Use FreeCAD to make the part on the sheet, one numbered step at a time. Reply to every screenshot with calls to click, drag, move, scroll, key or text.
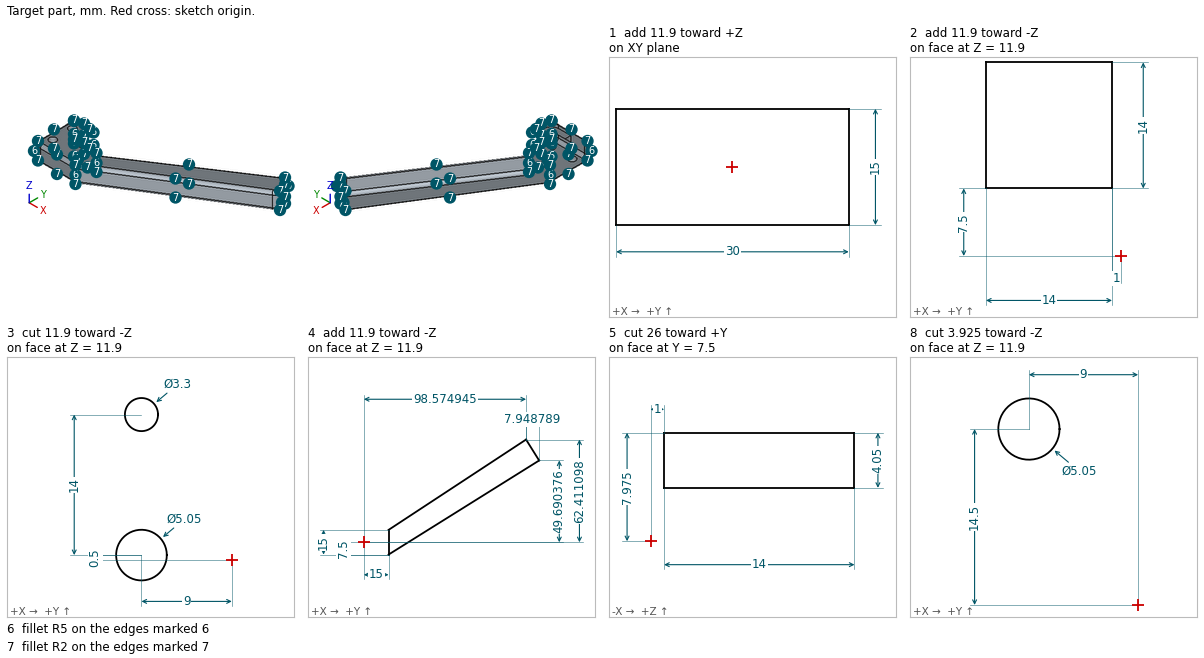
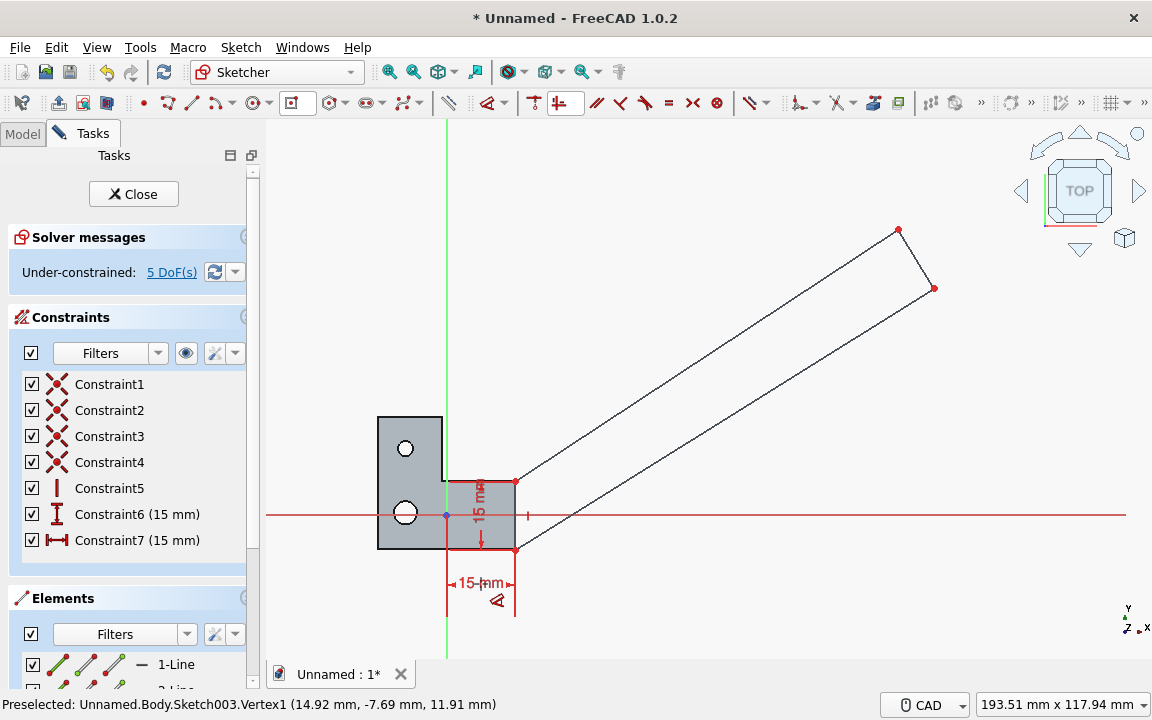
click(515, 550)
click(413, 533)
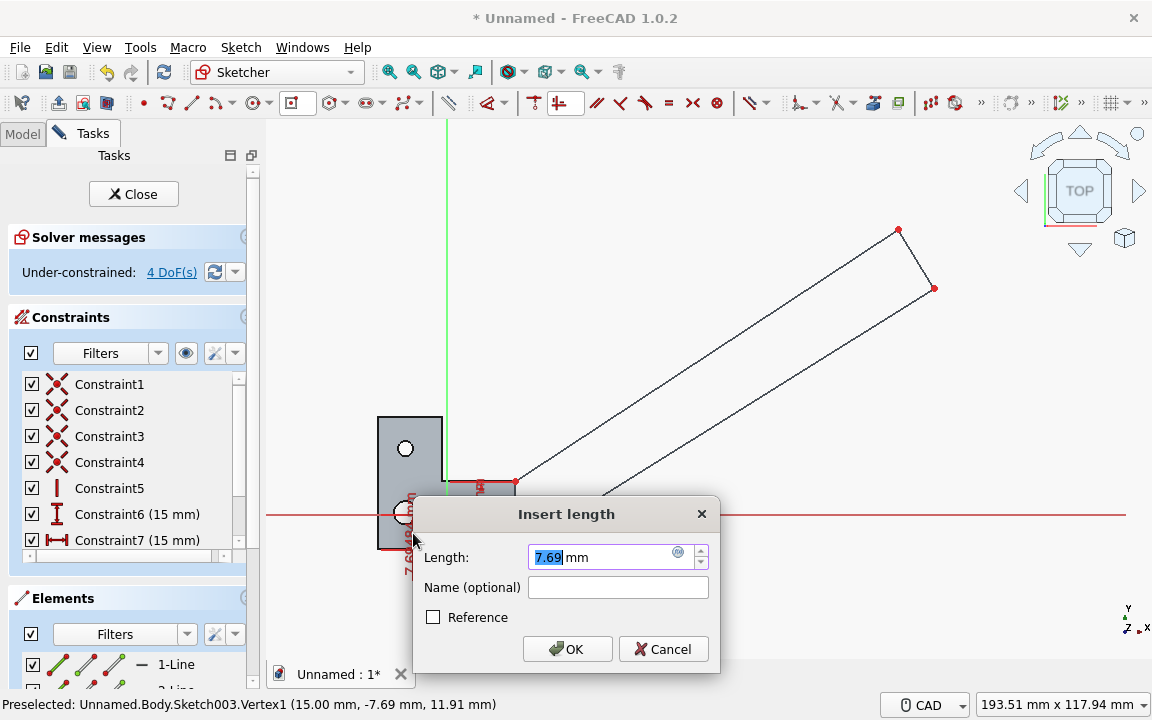
text(7.5)
key(Return)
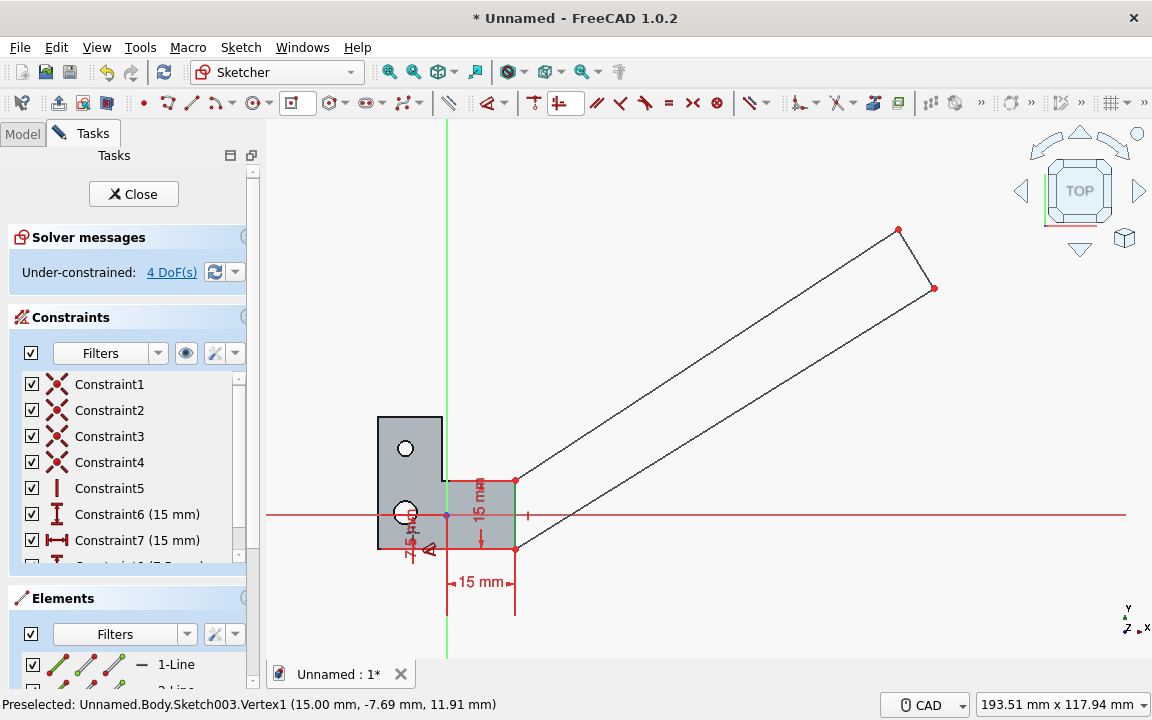
click(923, 271)
click(916, 196)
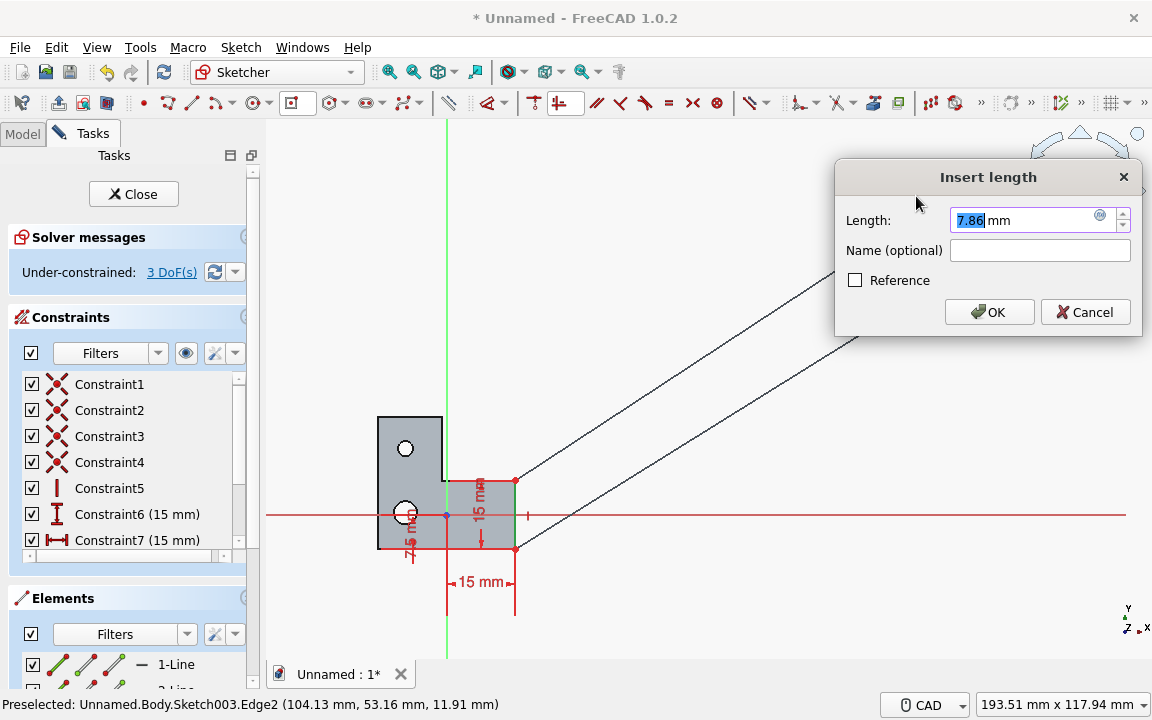
text(7.948789)
key(Return)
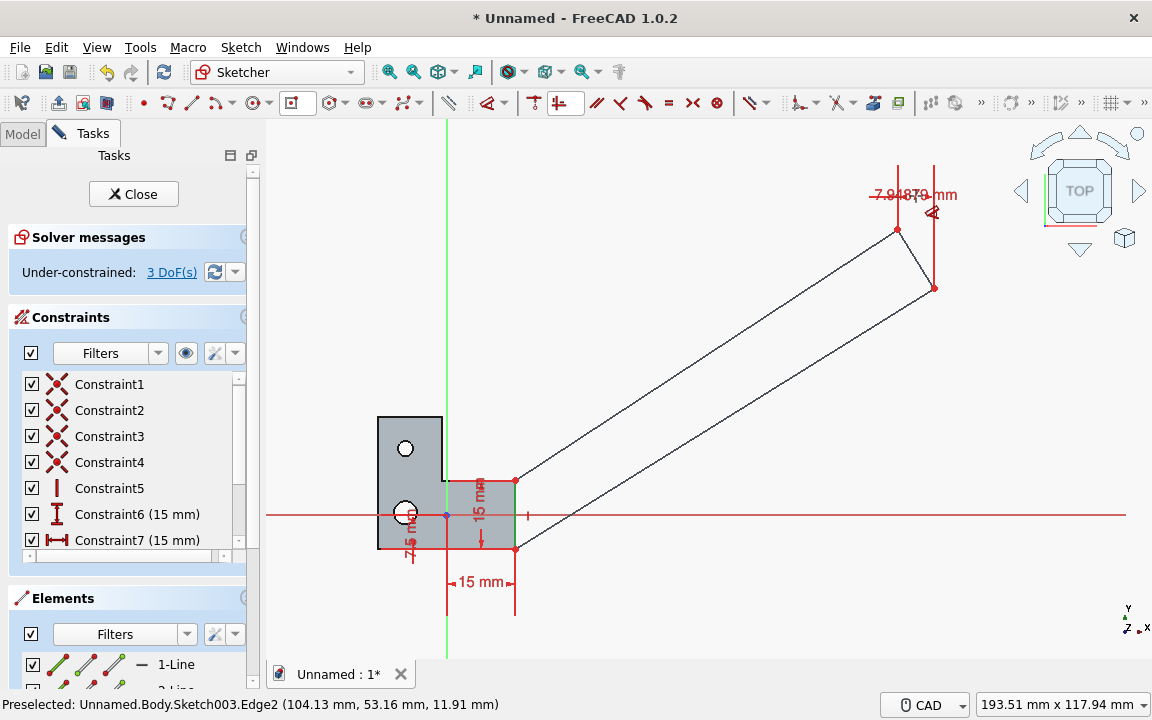
click(934, 289)
click(413, 402)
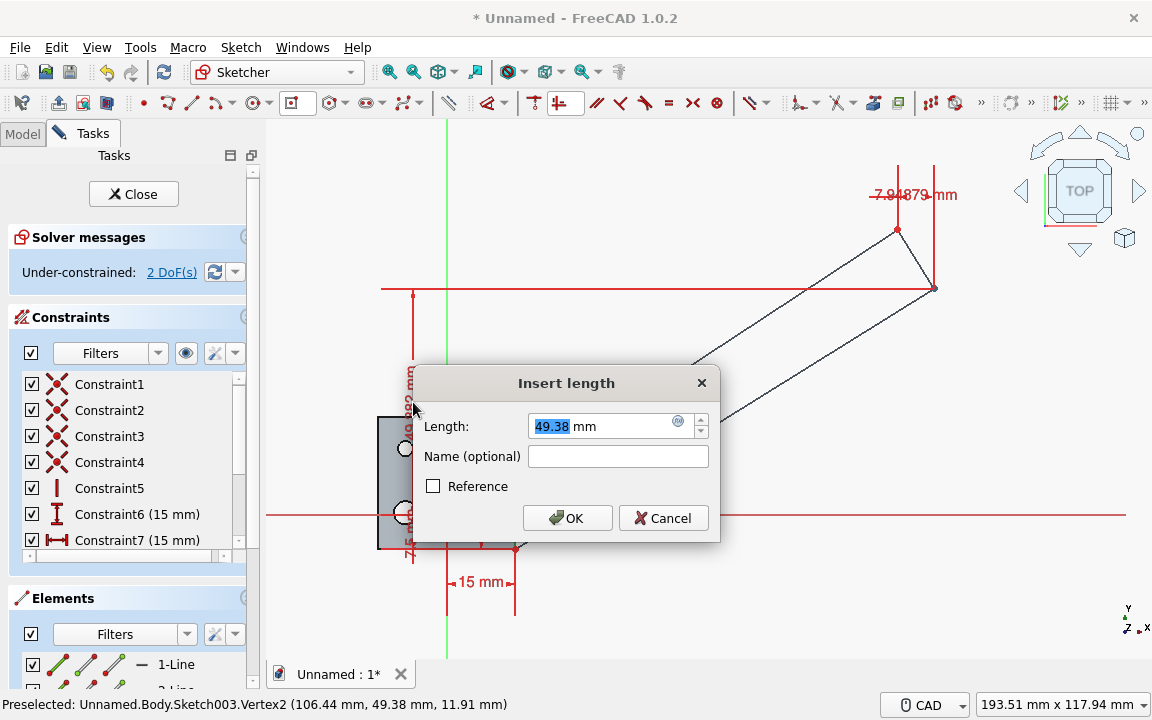
text(49.690376)
key(Return)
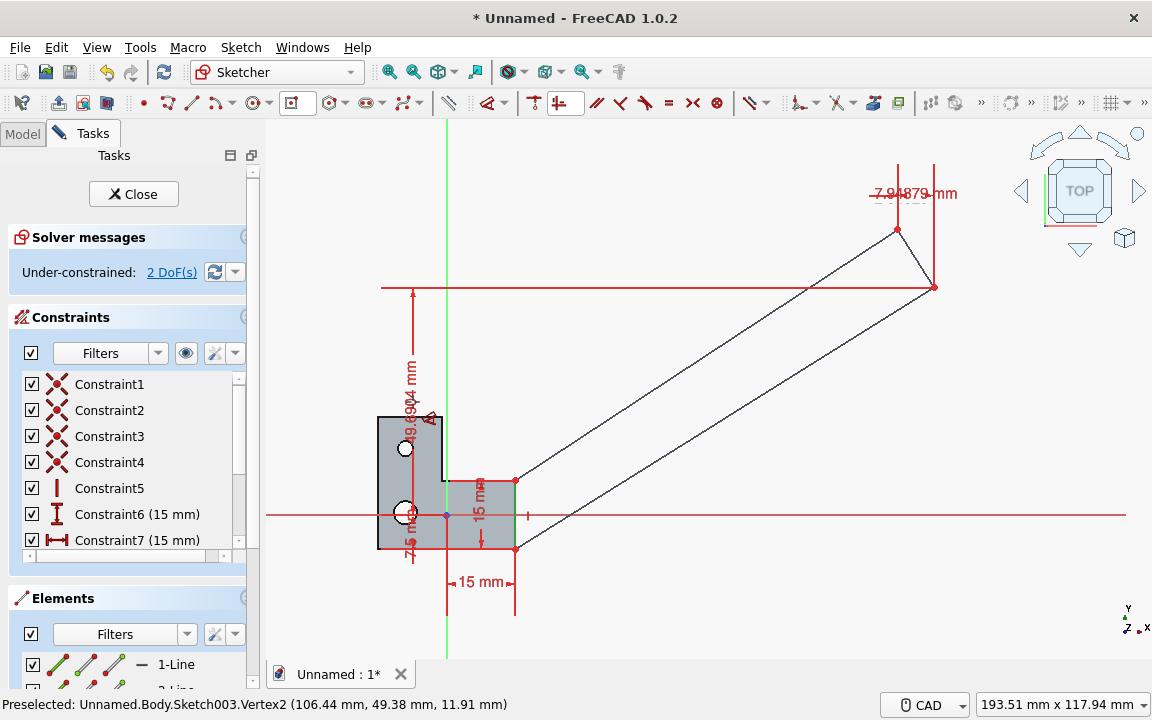
click(898, 230)
click(672, 196)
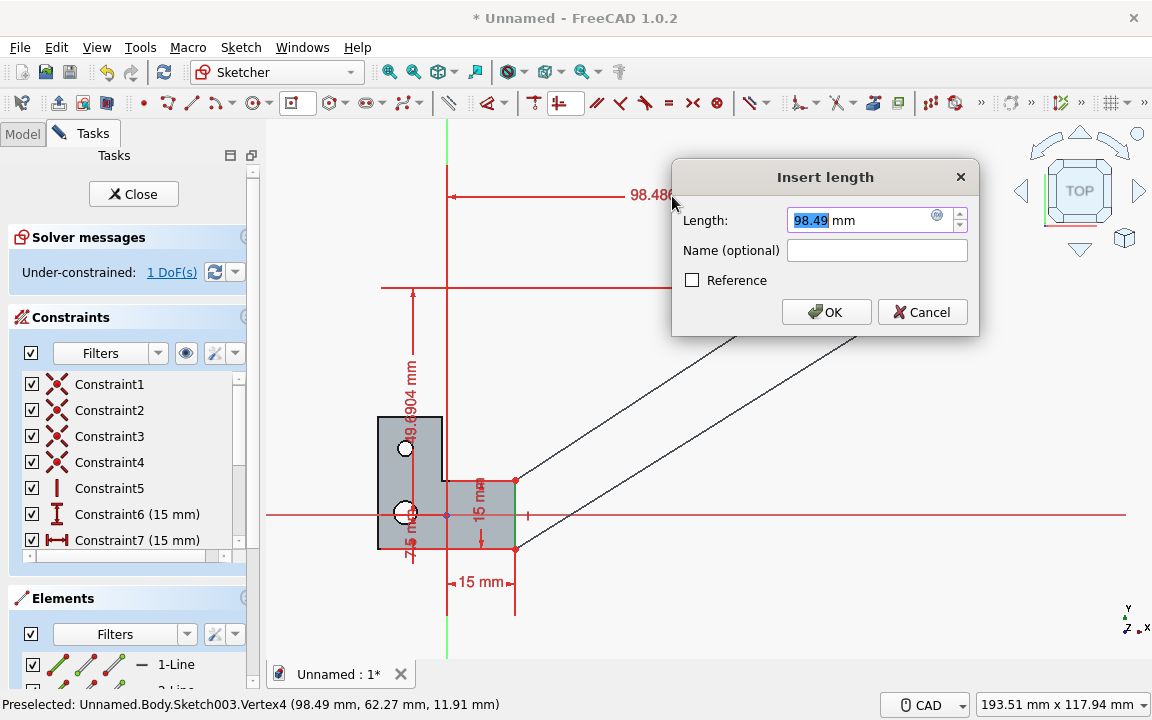
text(98.574945)
key(Return)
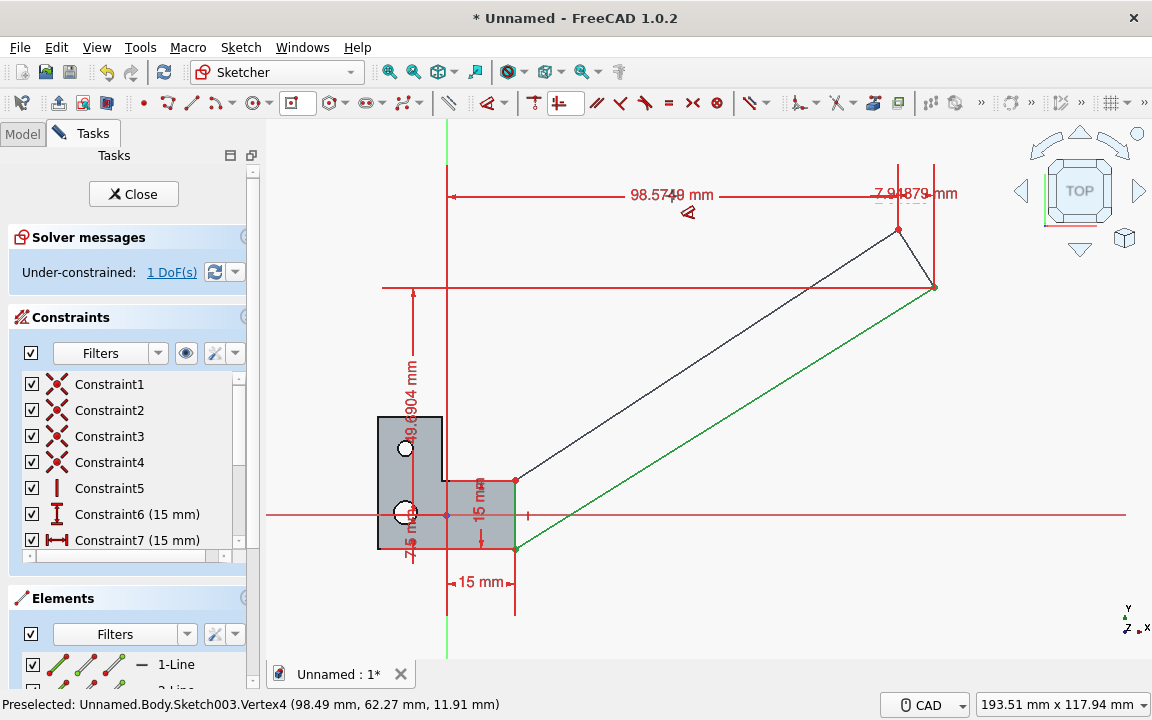
click(898, 230)
click(413, 373)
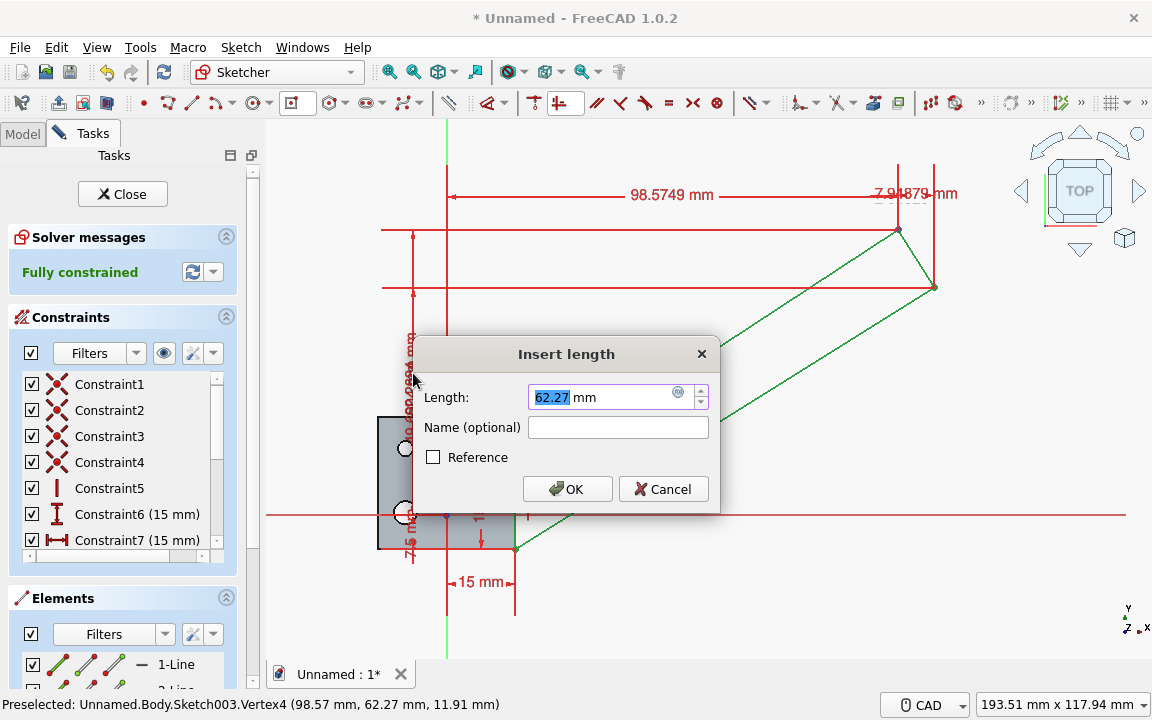
text(62.411098)
key(Return)
key(Escape)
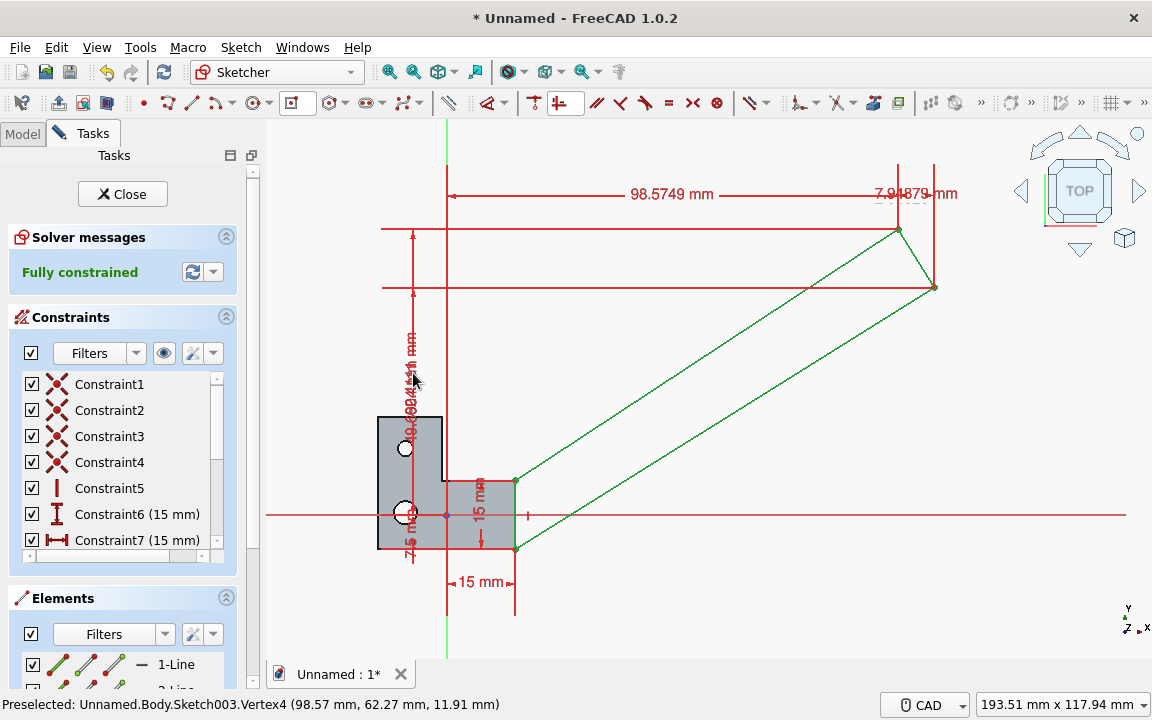
click(123, 194)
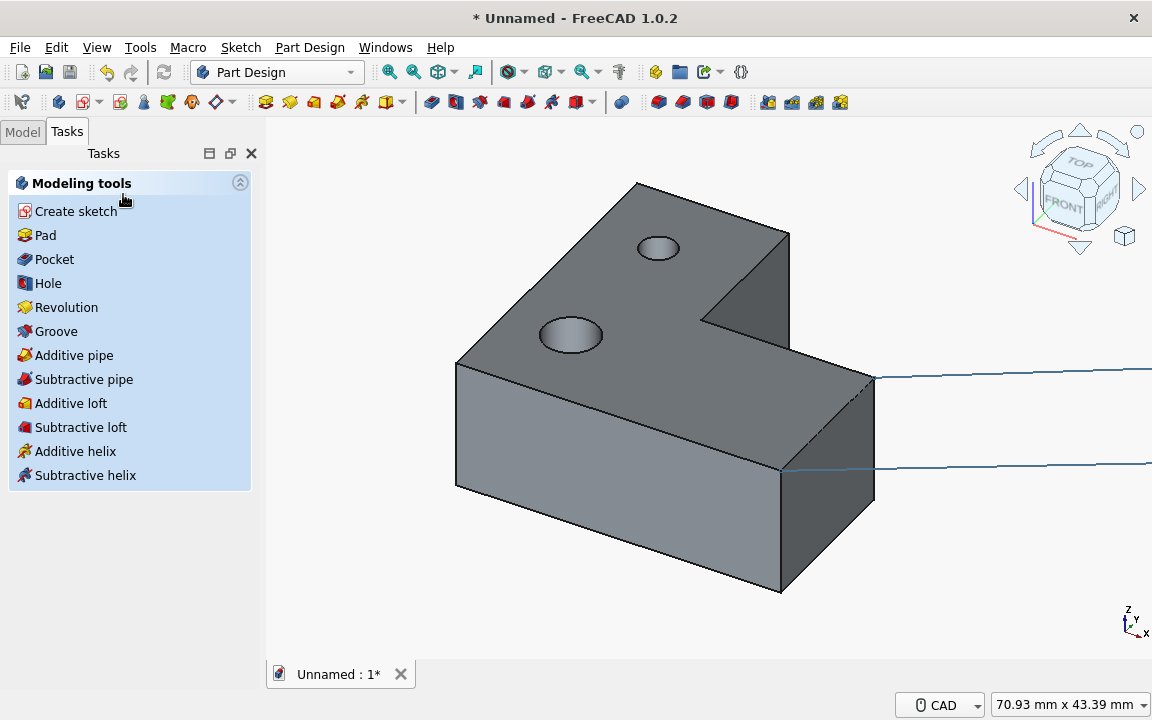
click(266, 102)